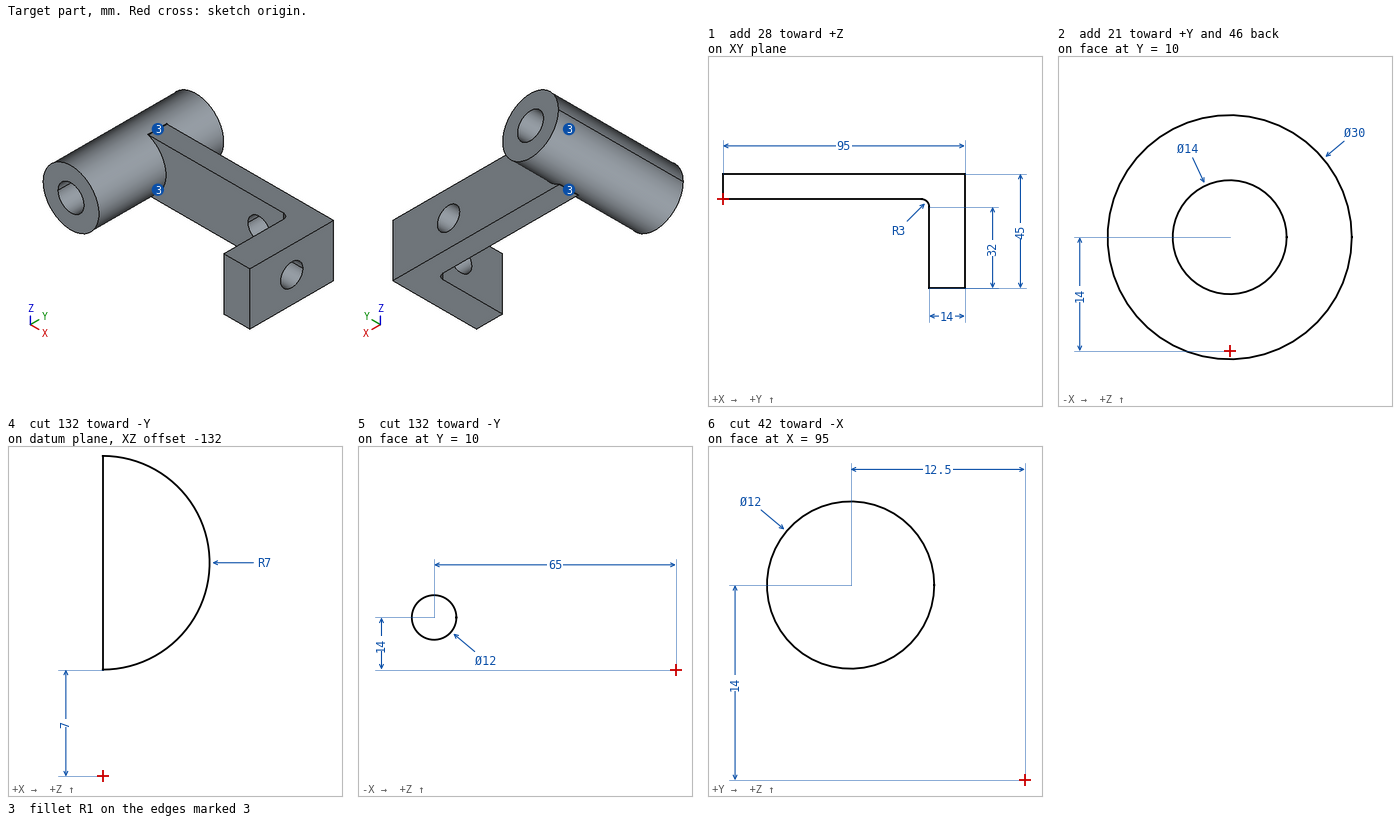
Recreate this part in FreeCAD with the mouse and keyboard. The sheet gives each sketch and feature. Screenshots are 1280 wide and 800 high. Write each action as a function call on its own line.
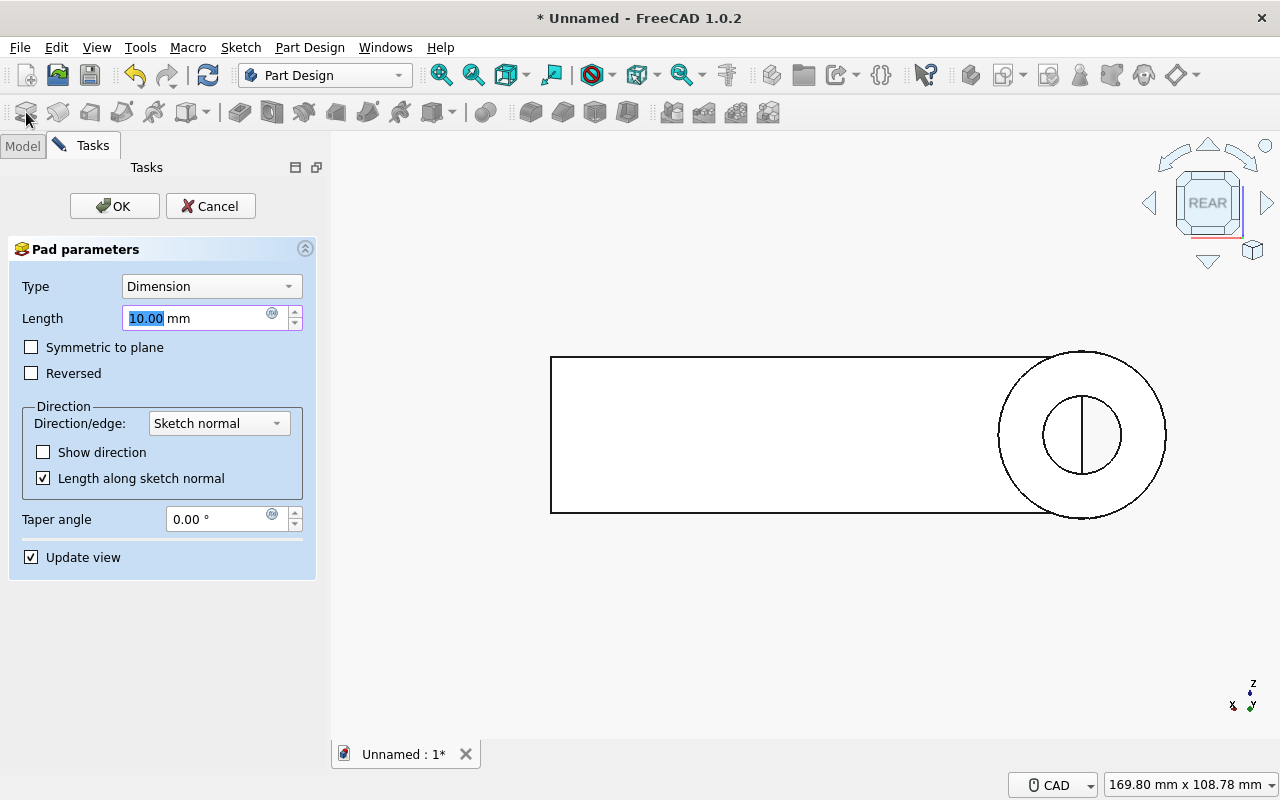
click(212, 286)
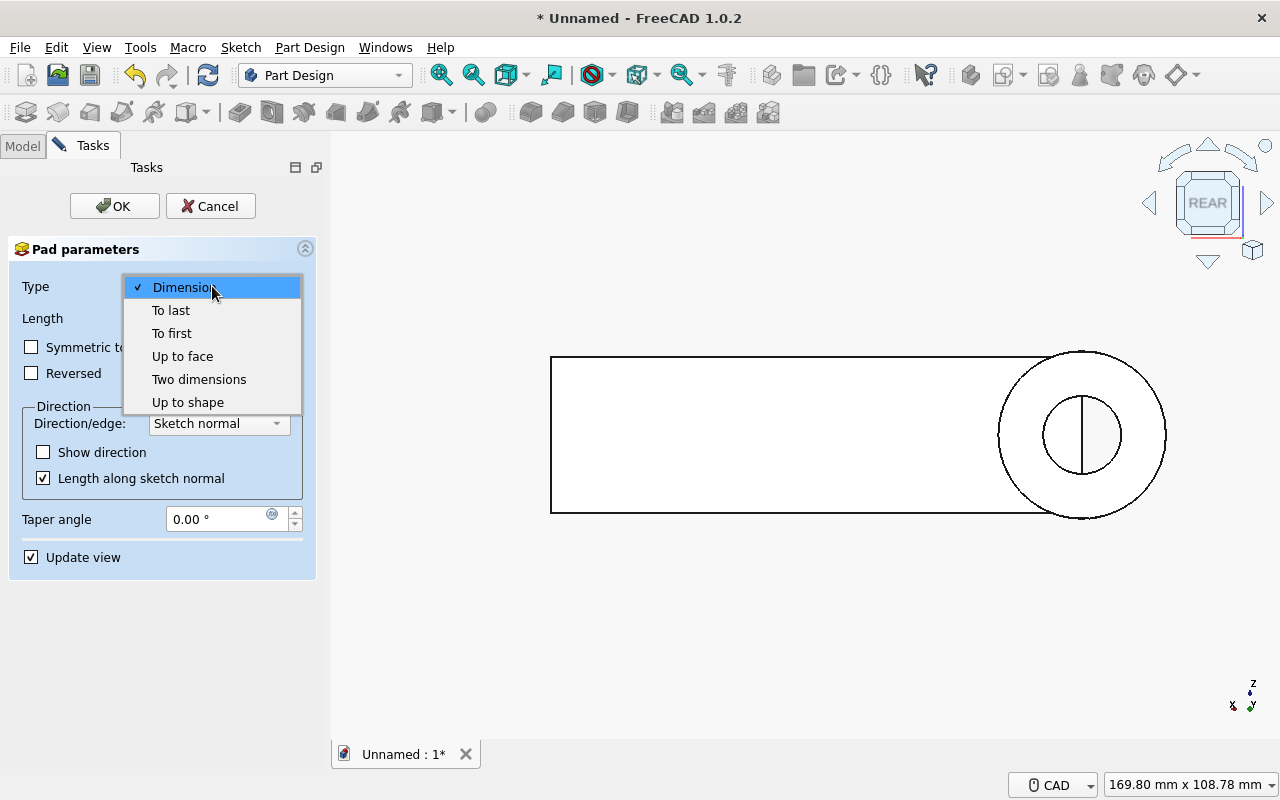
click(212, 380)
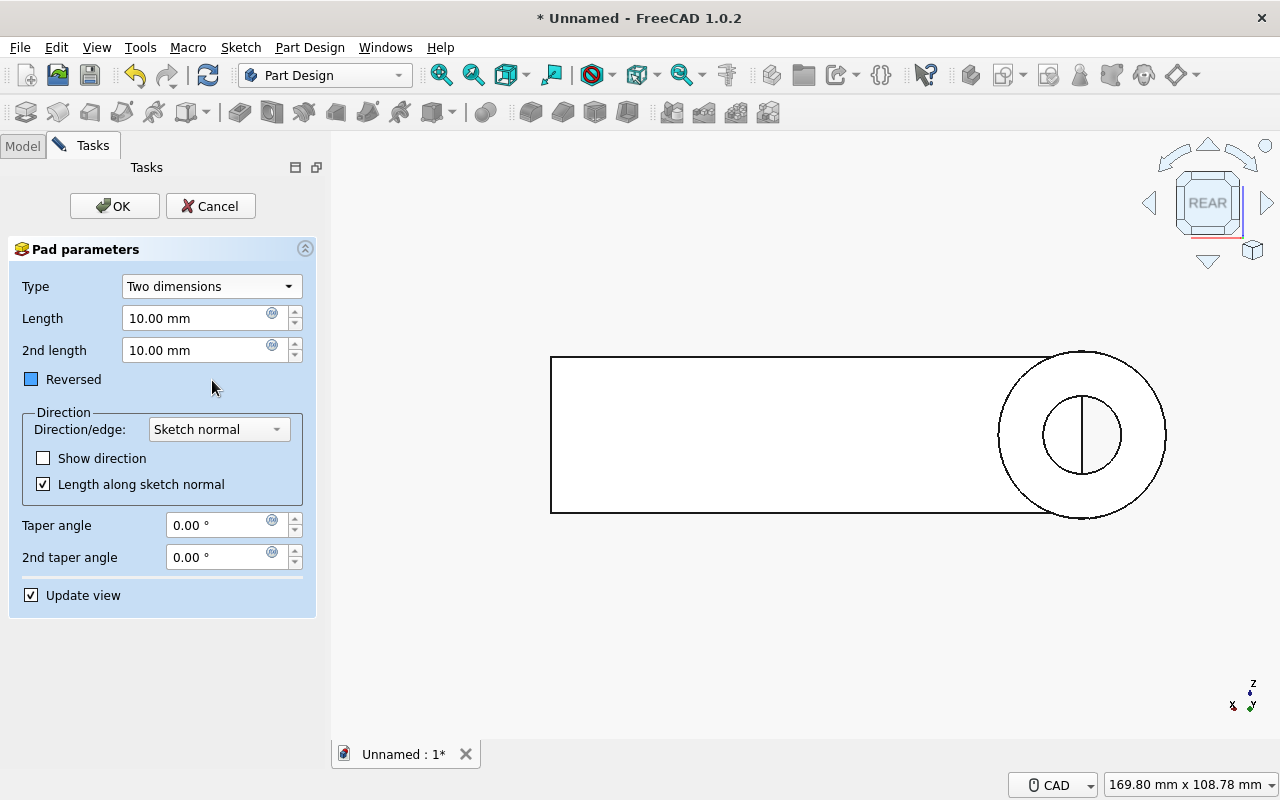
triple_click(204, 318)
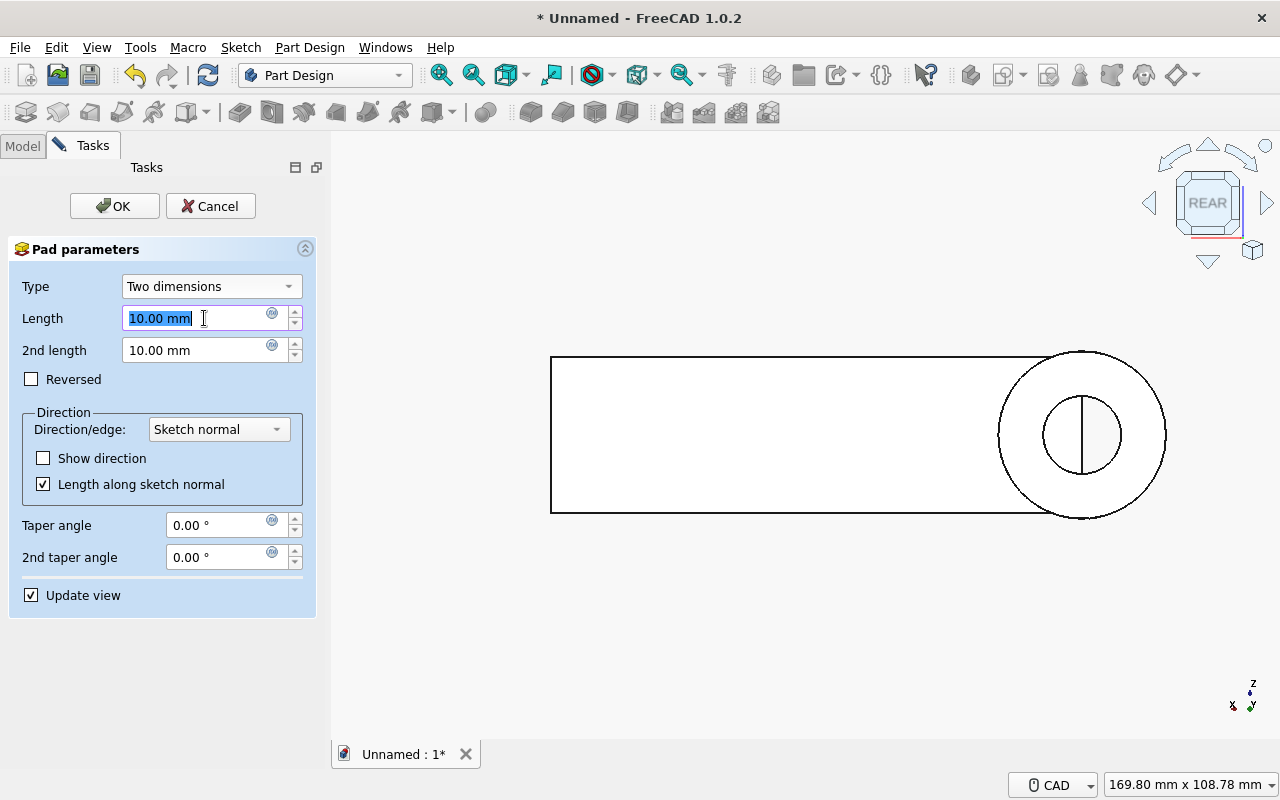
text(21)
key(Tab)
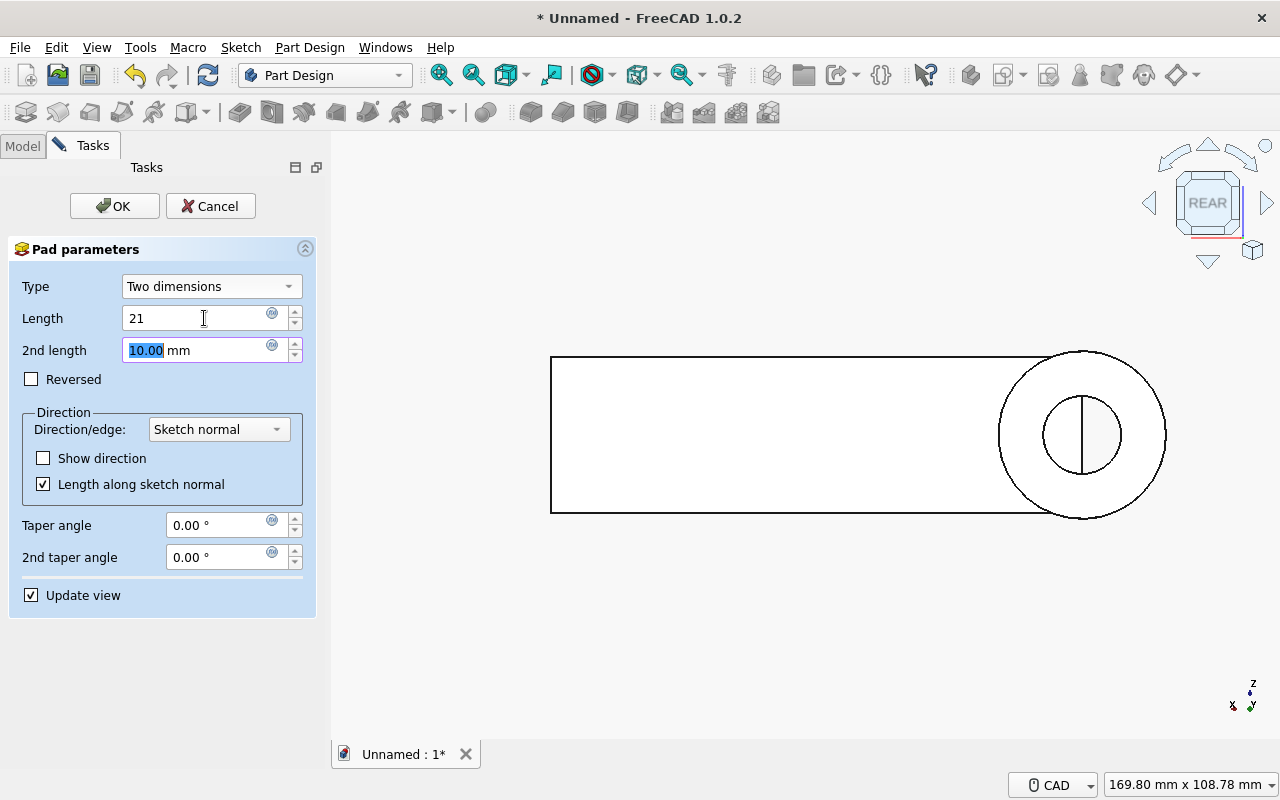
text(46)
key(Tab)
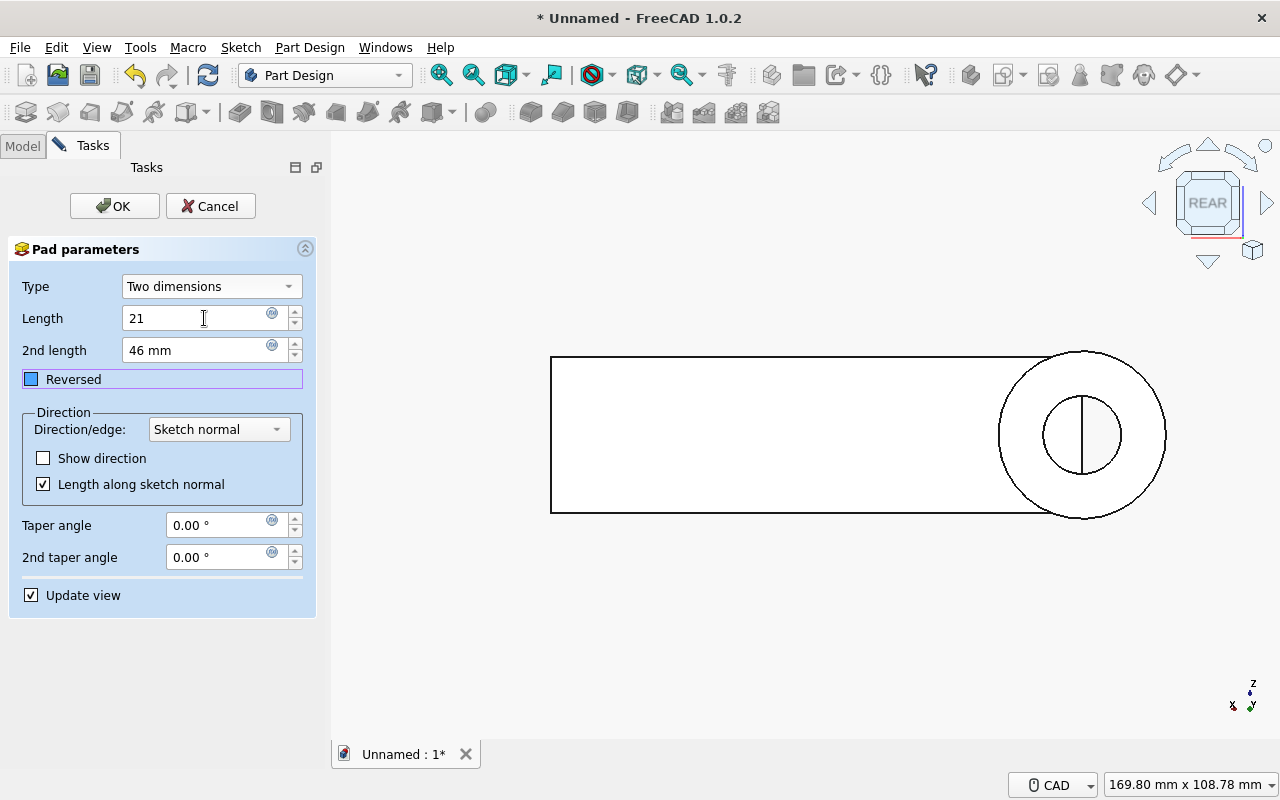
click(115, 206)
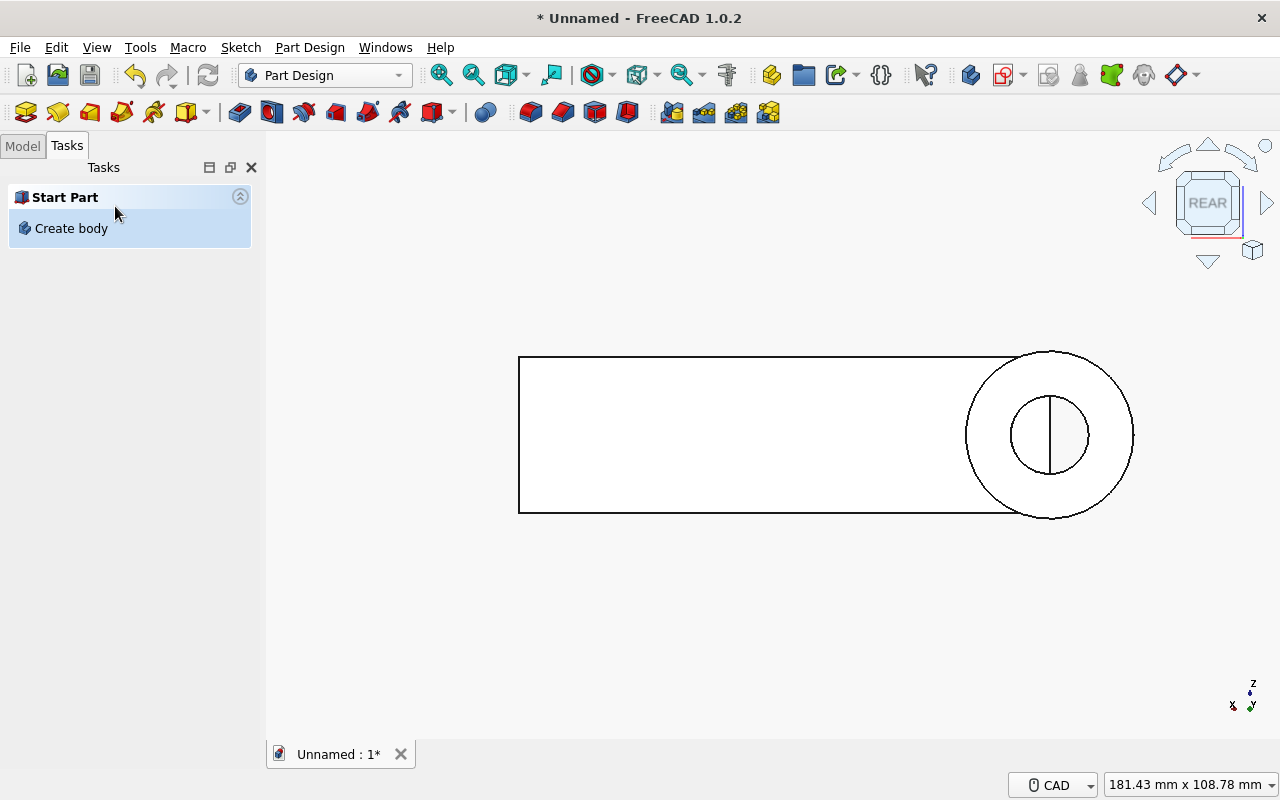
key(0)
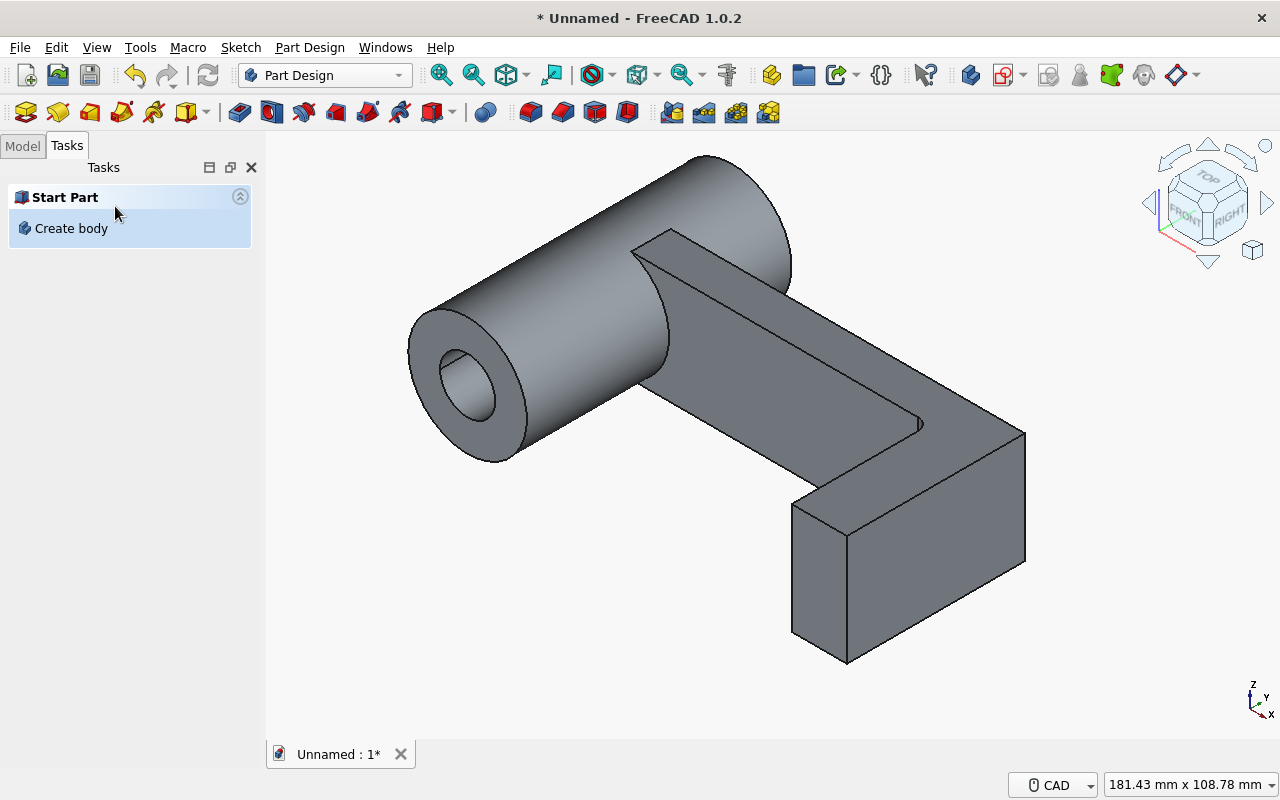
click(442, 76)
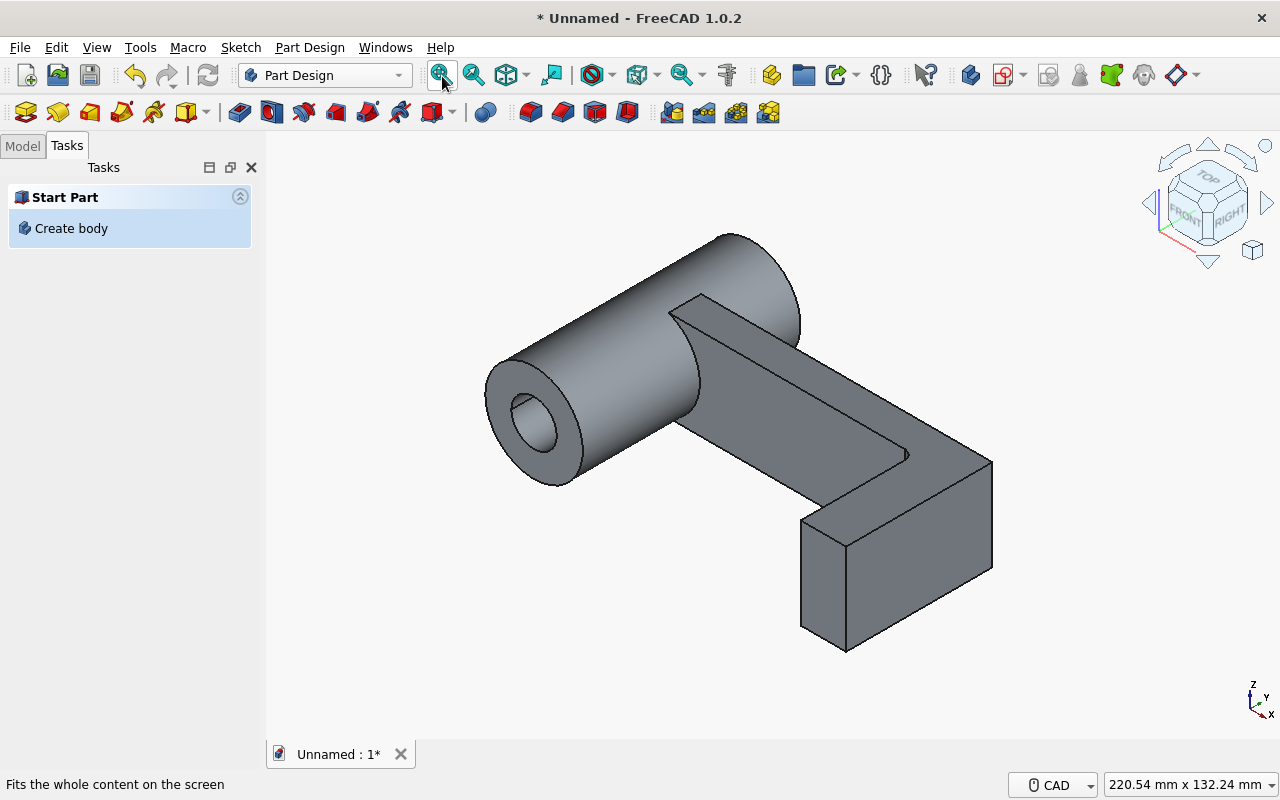
key(2)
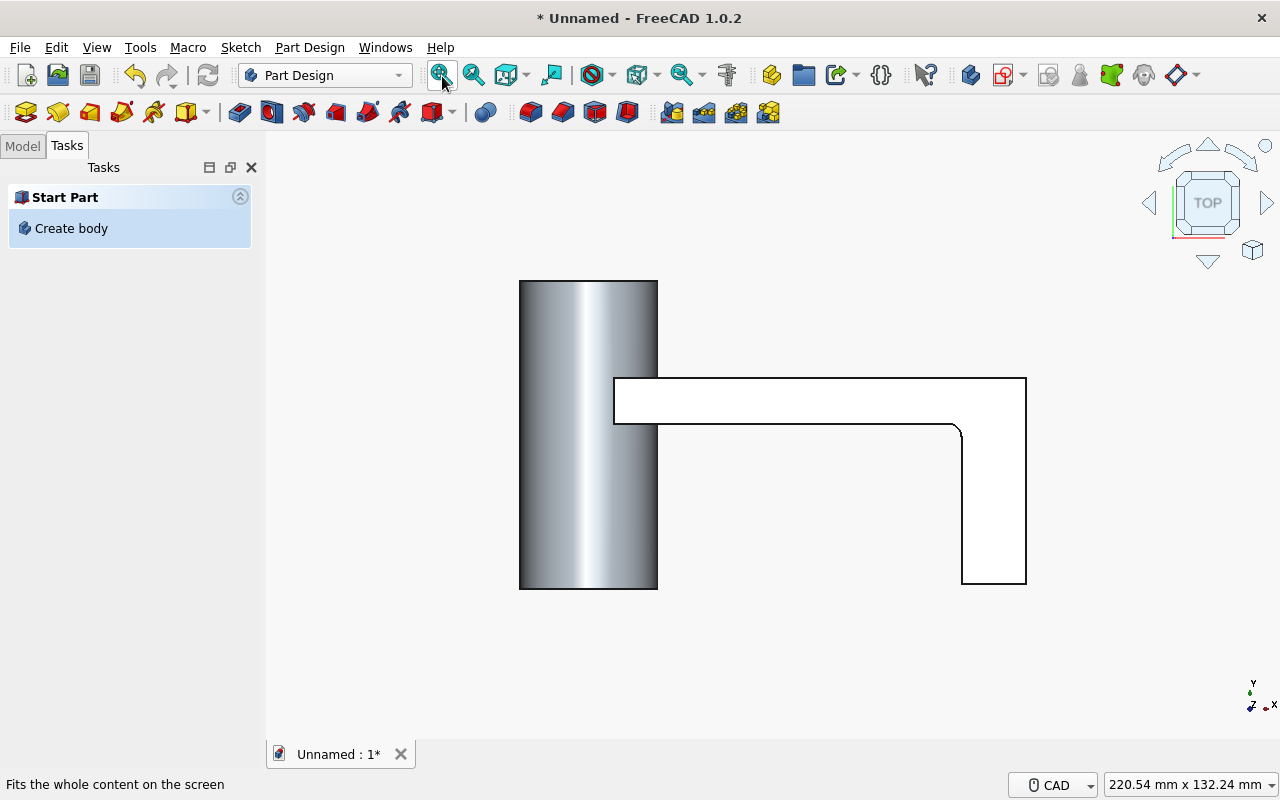
key(1)